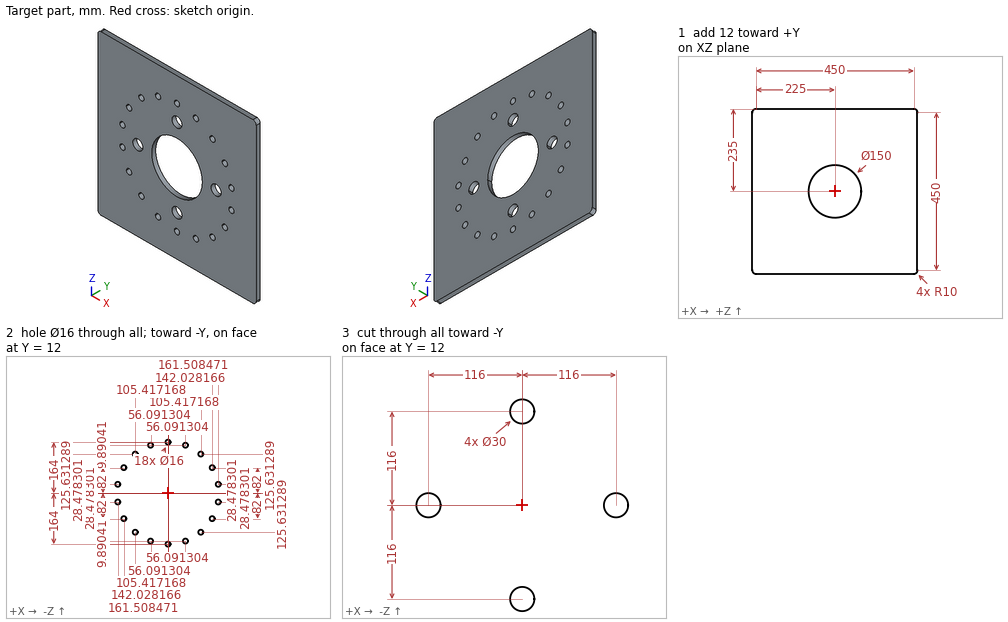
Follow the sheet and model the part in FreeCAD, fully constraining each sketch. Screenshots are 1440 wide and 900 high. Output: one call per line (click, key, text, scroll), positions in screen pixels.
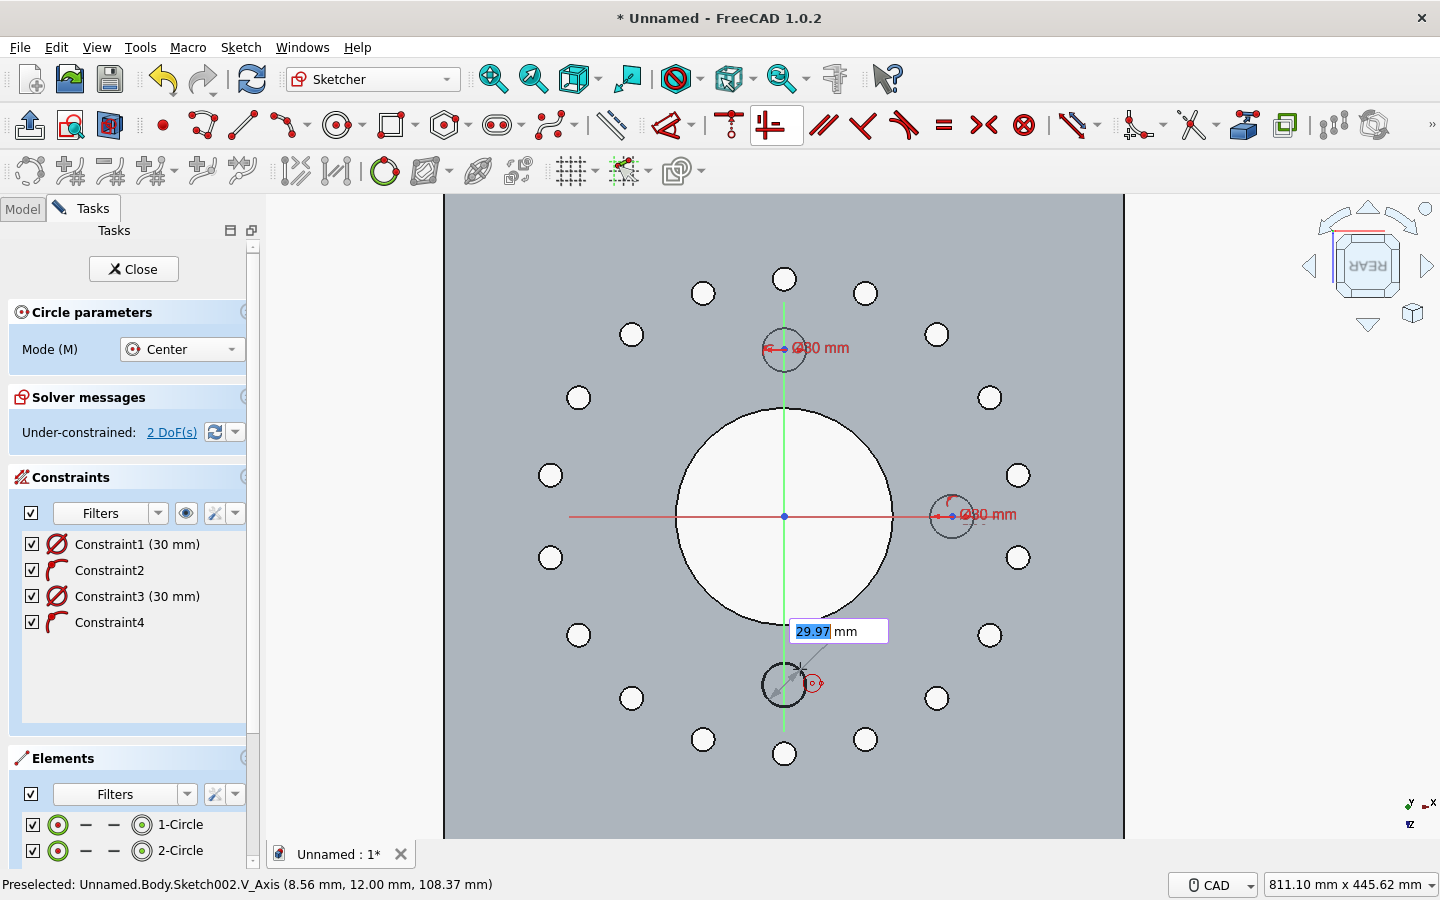
text(30)
key(Return)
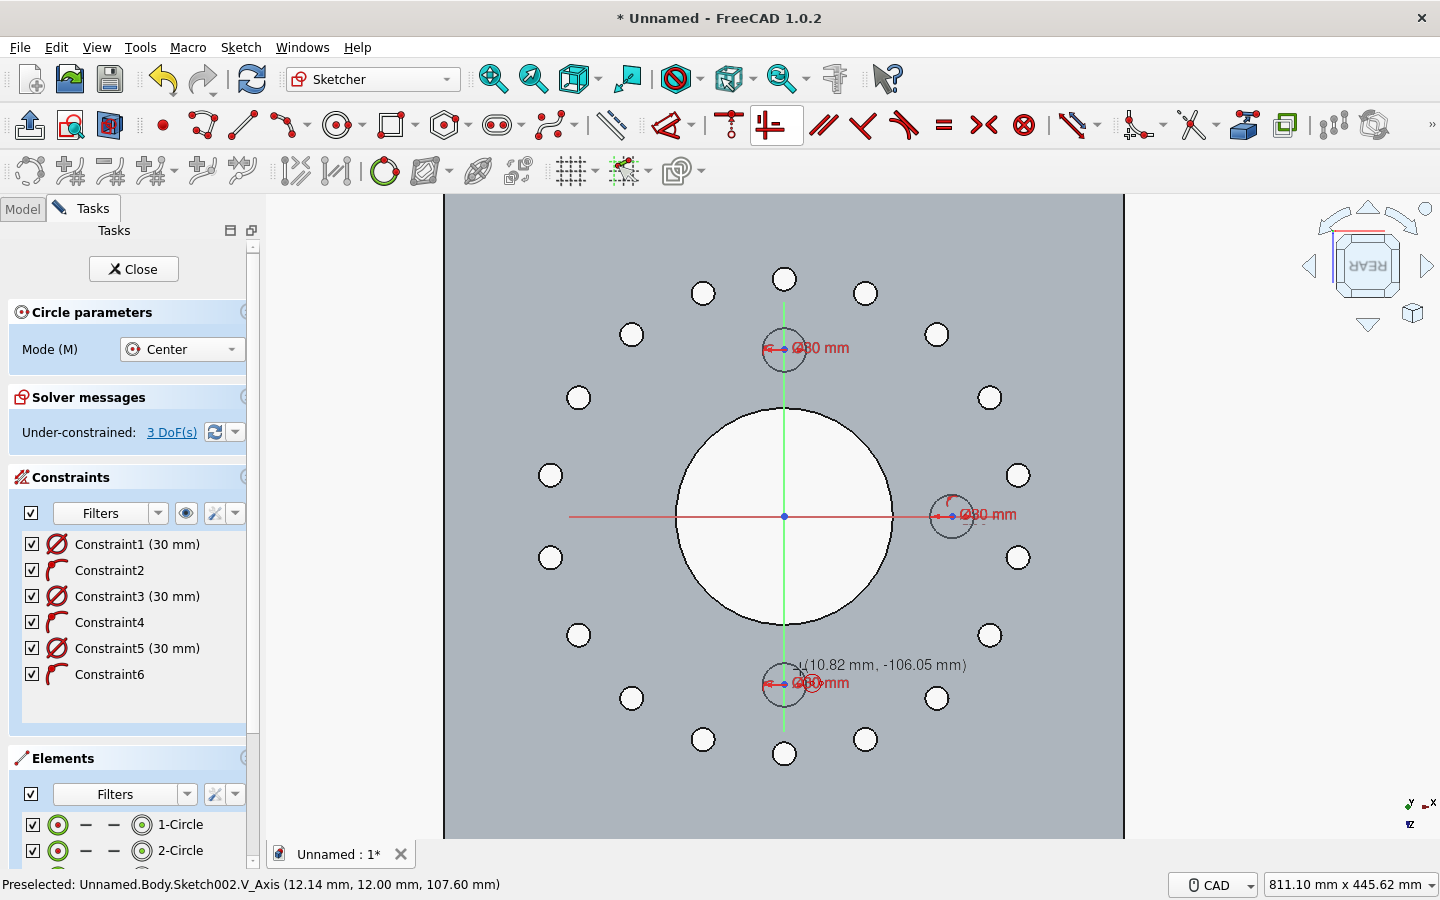
click(616, 516)
move(632, 501)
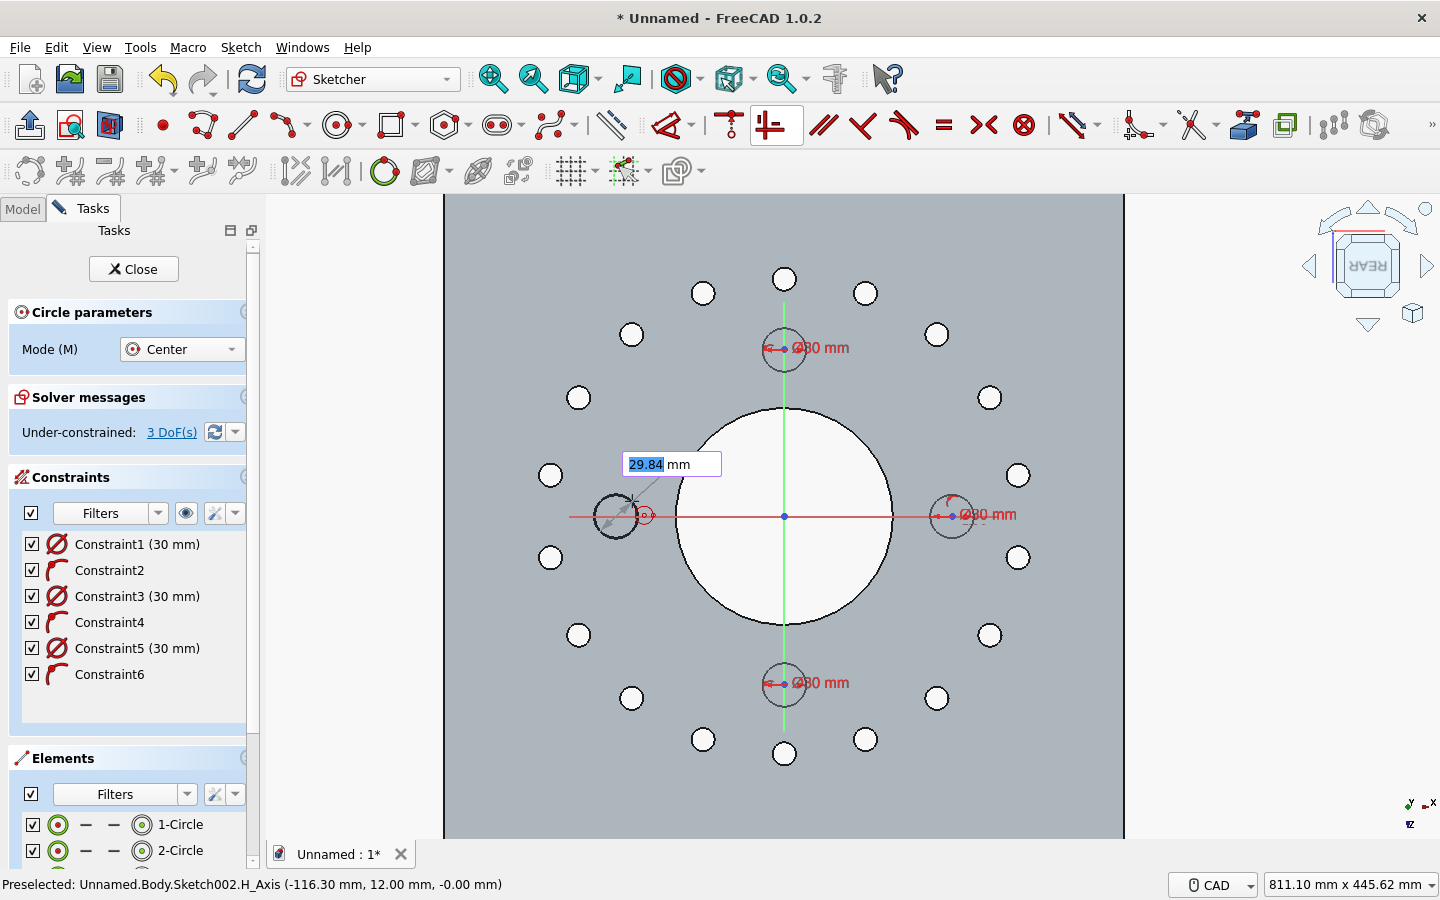
text(30)
key(Return)
key(Escape)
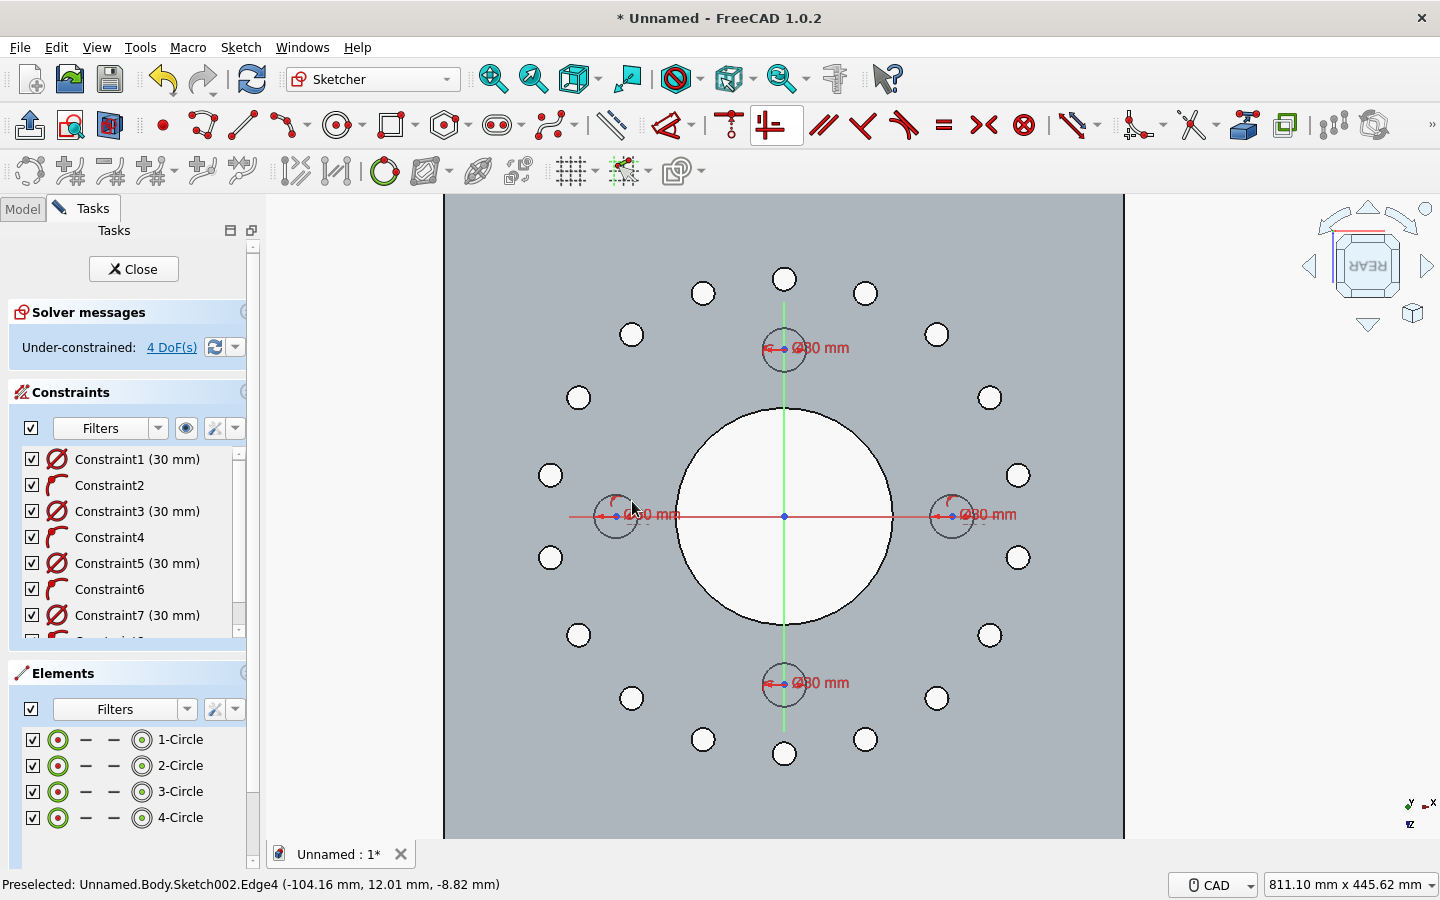
click(666, 126)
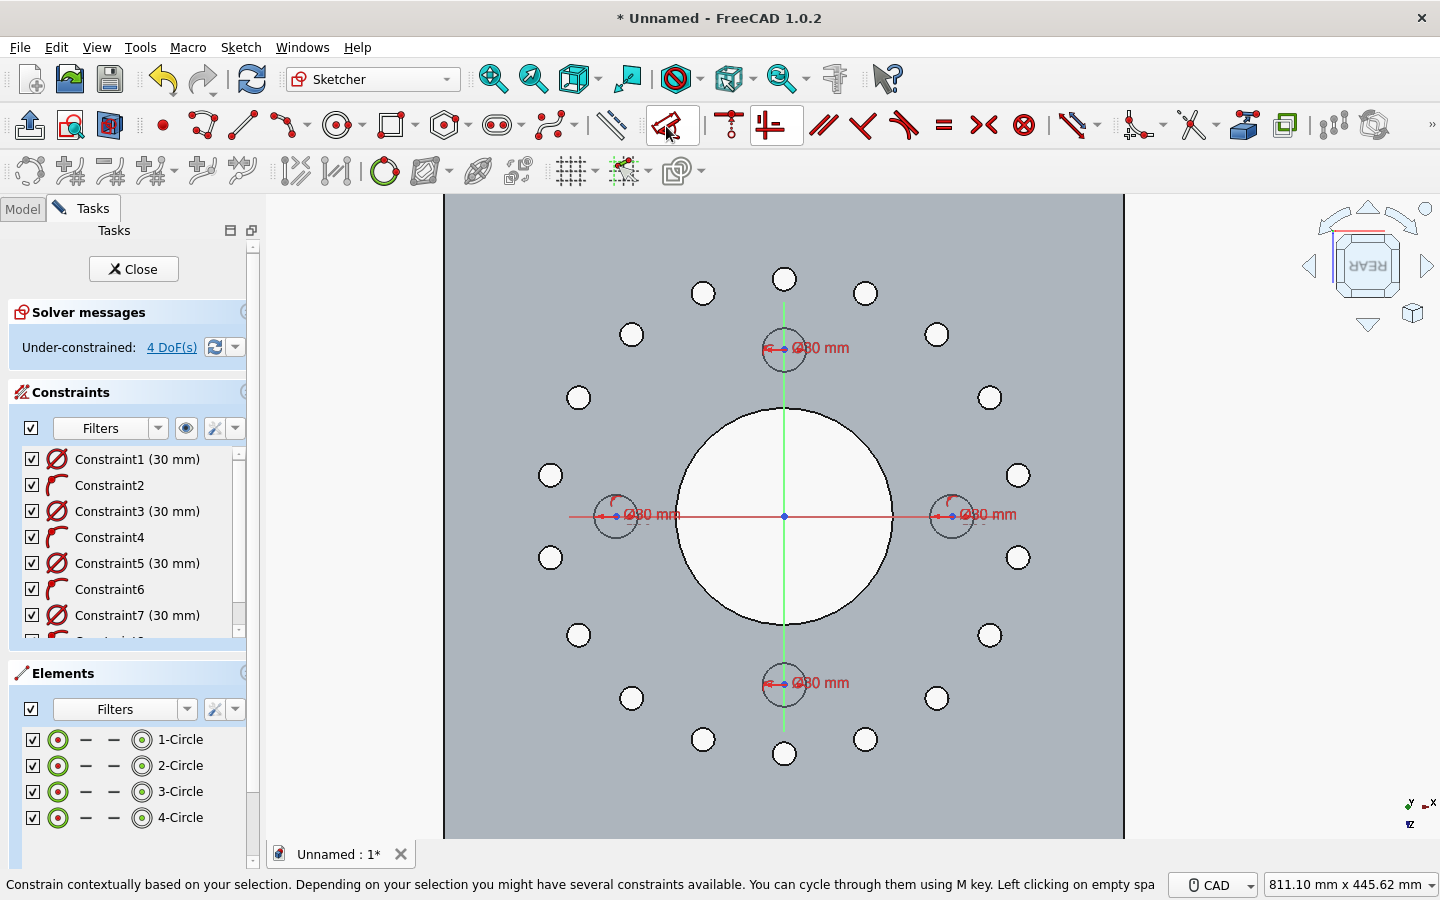
click(784, 350)
click(818, 433)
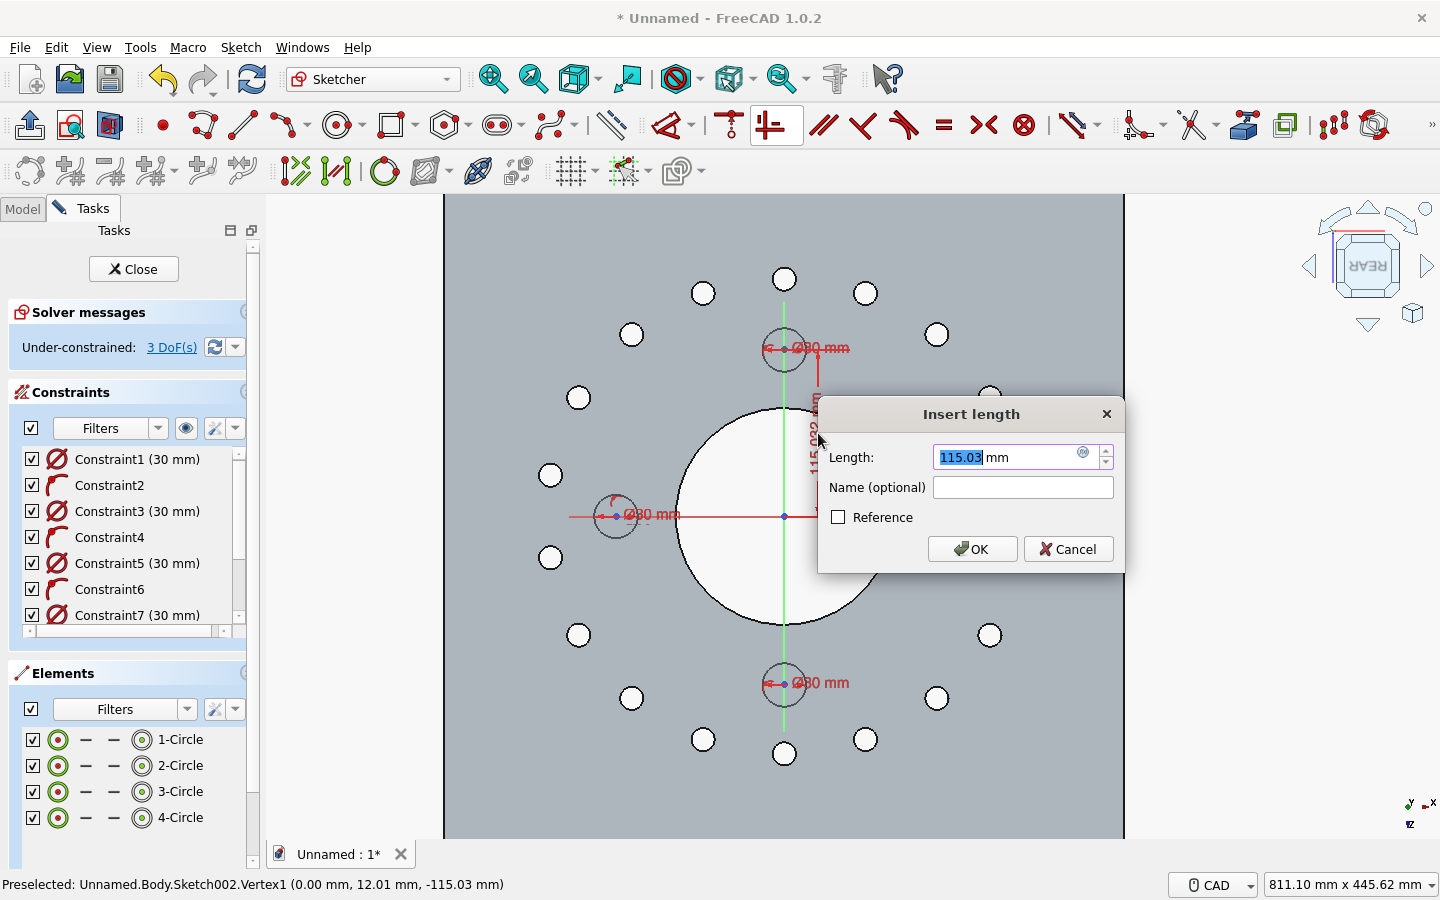
text(116)
key(Return)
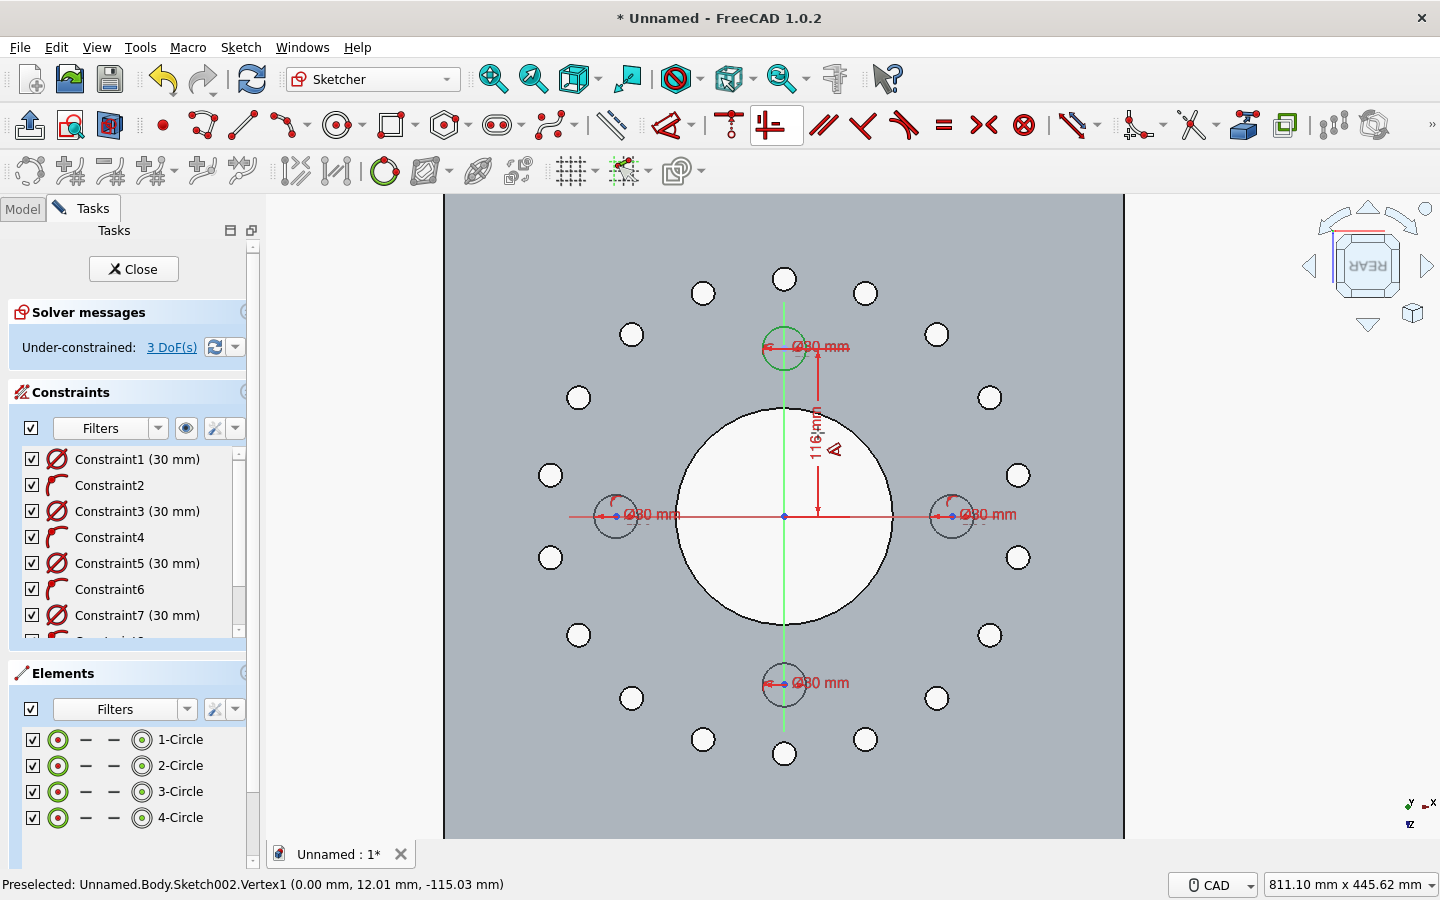
click(952, 516)
click(868, 550)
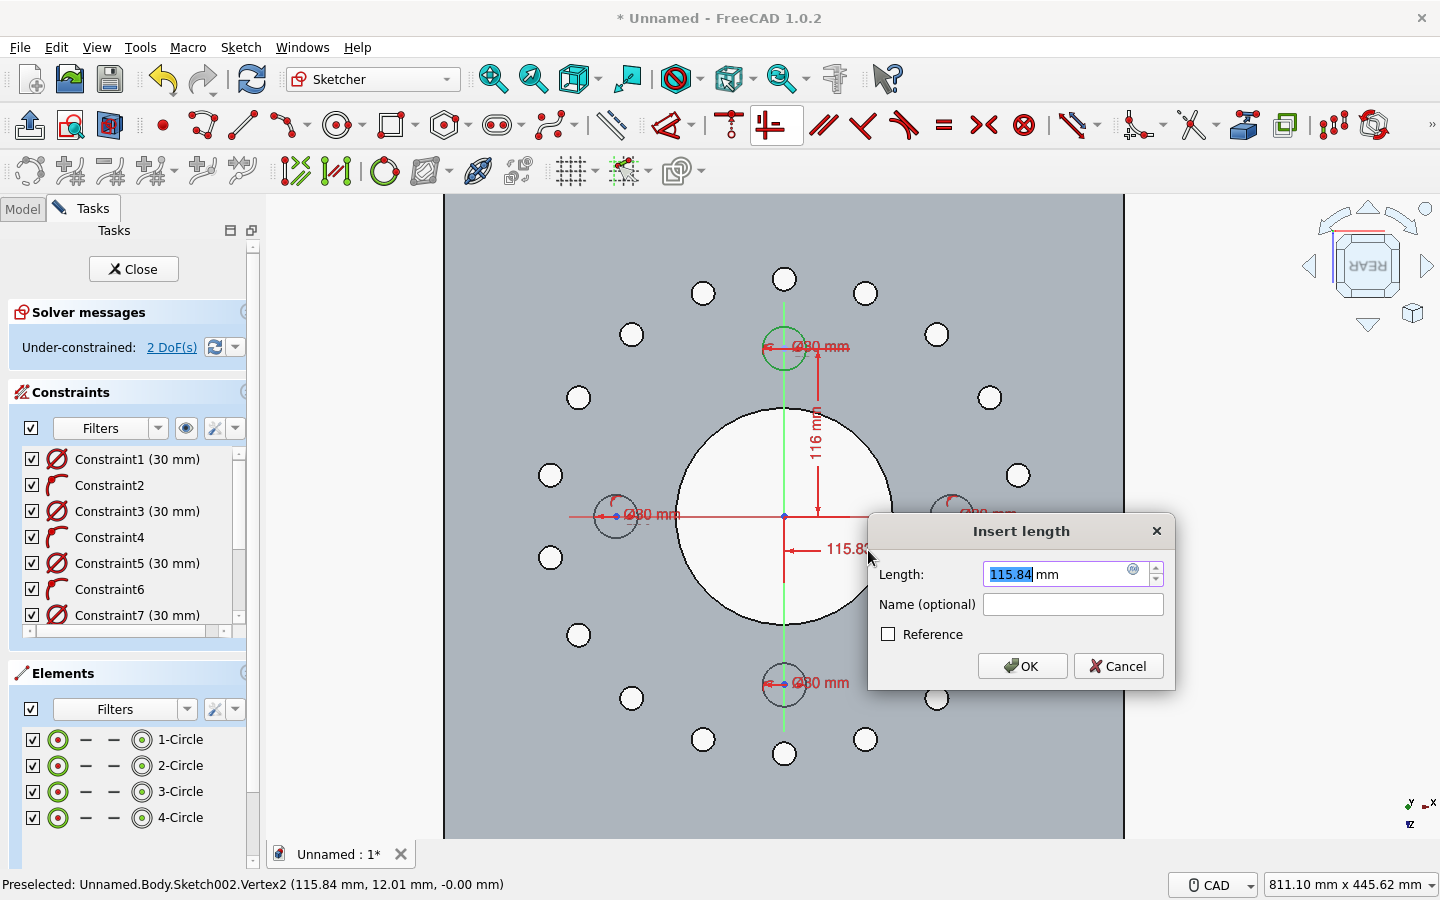
text(116)
key(Return)